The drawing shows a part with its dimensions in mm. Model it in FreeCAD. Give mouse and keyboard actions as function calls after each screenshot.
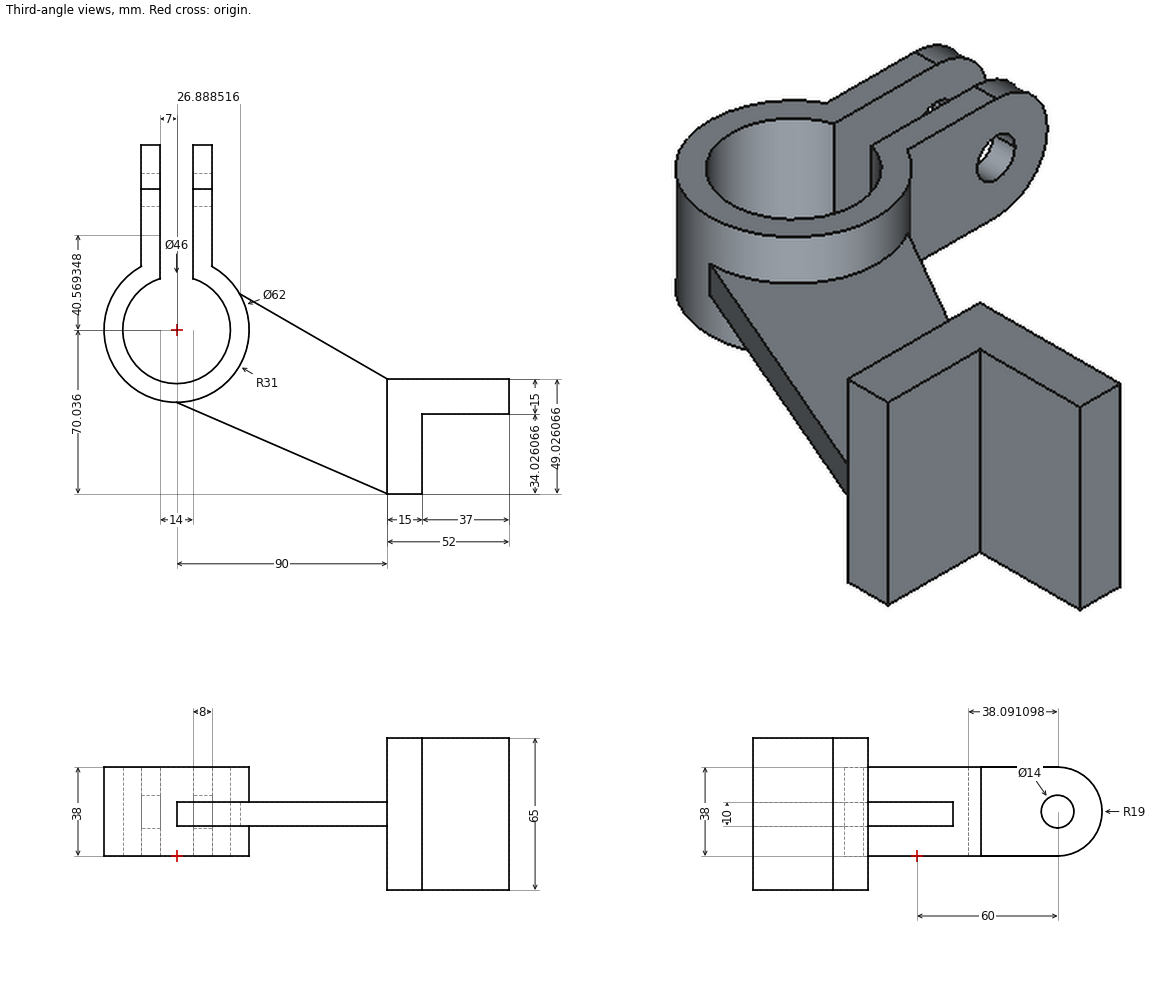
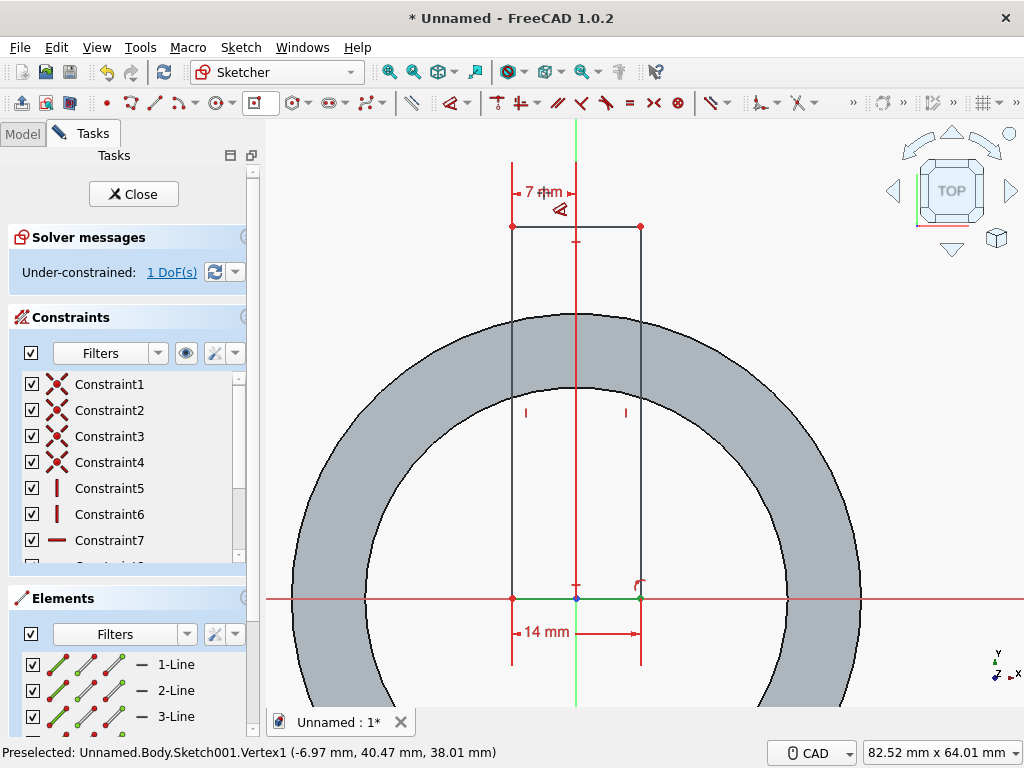
click(512, 339)
click(478, 413)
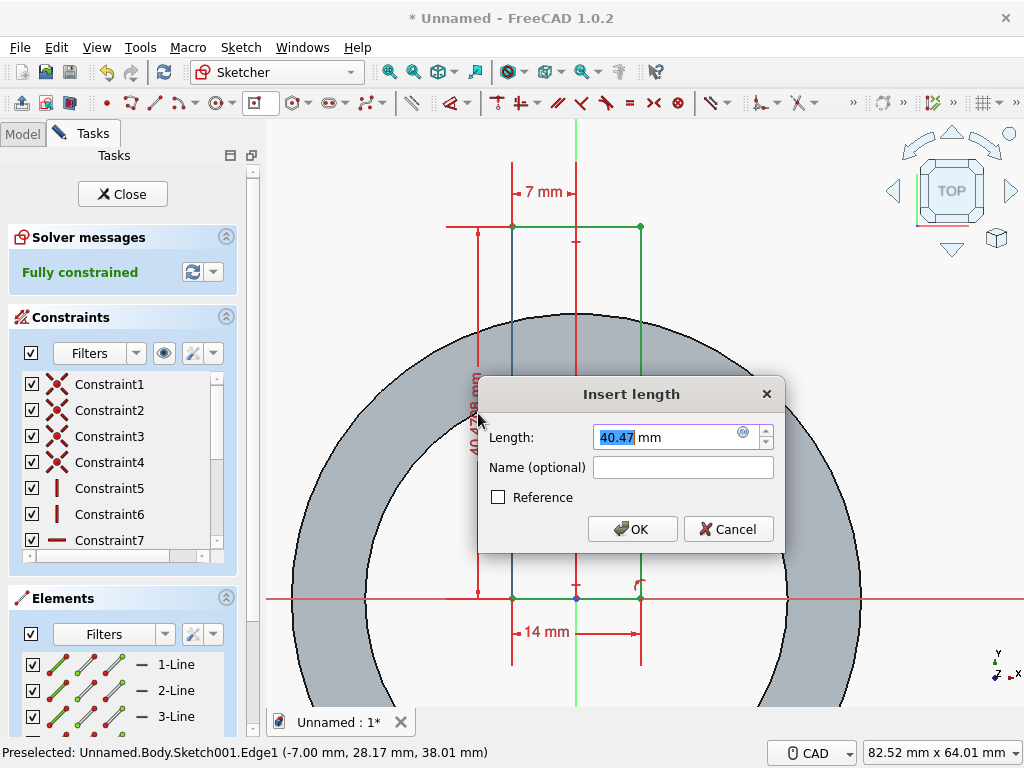
text(40.569348)
key(Return)
key(Escape)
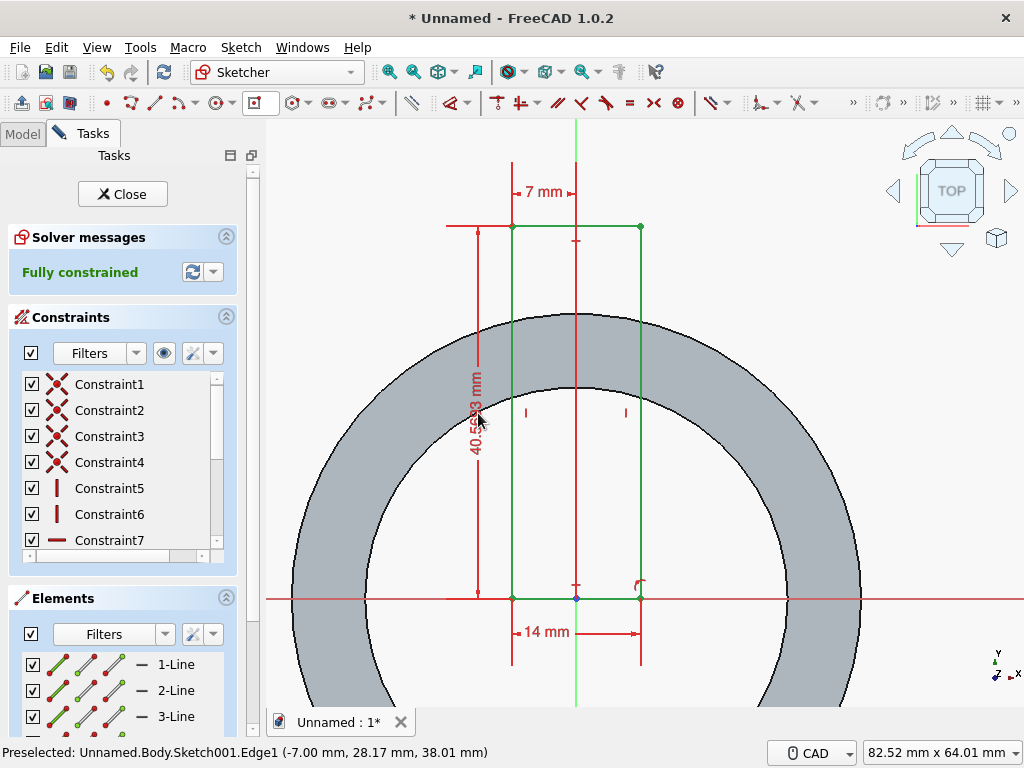
click(123, 194)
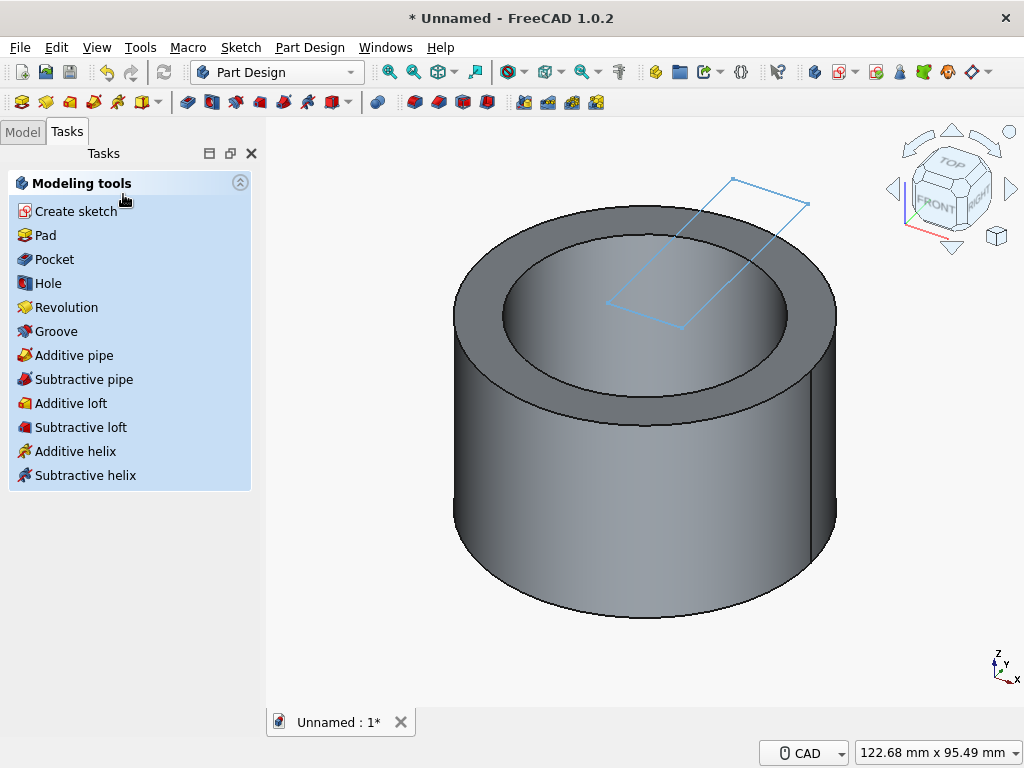
click(188, 102)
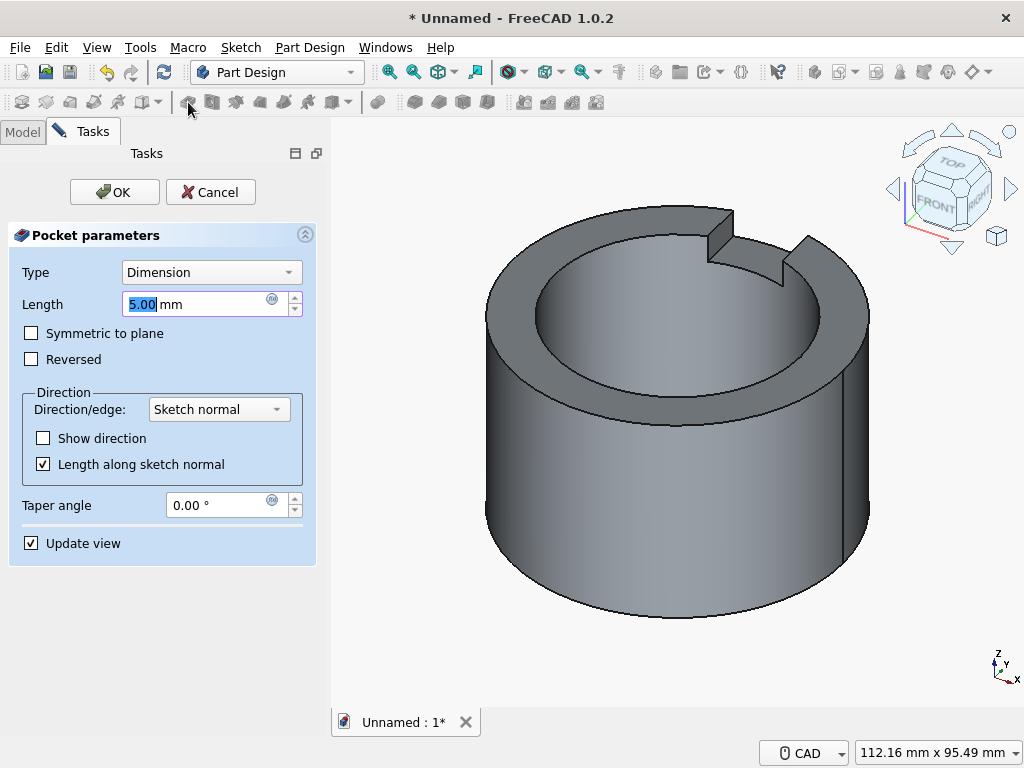
text(38)
key(Tab)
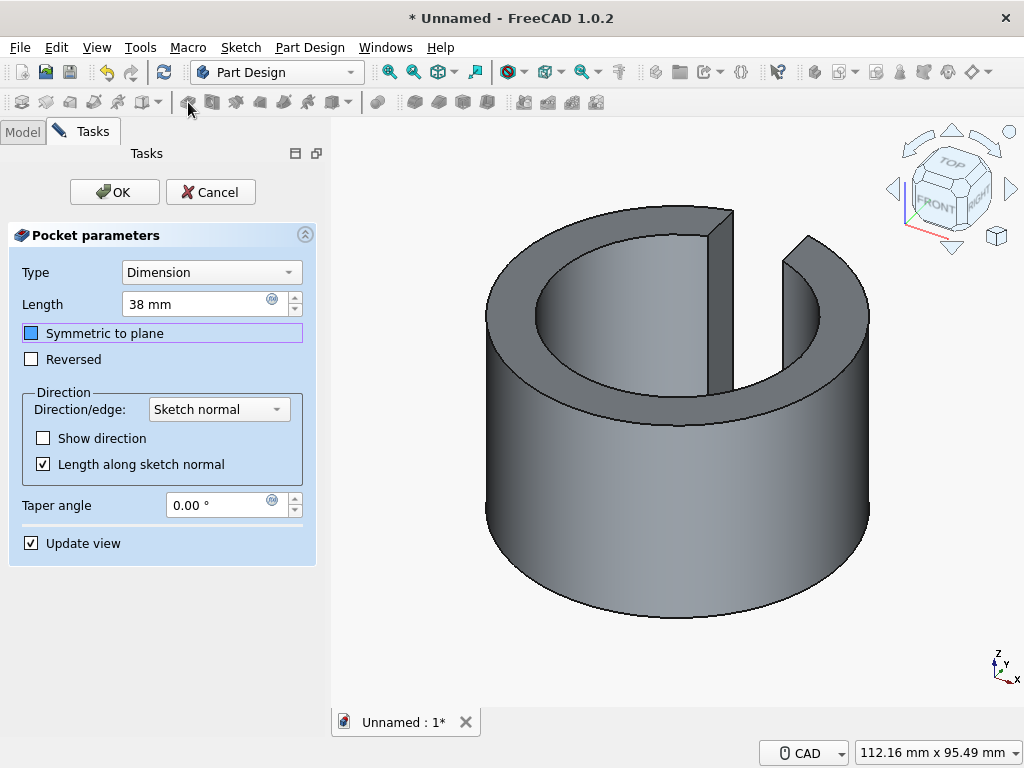
click(115, 192)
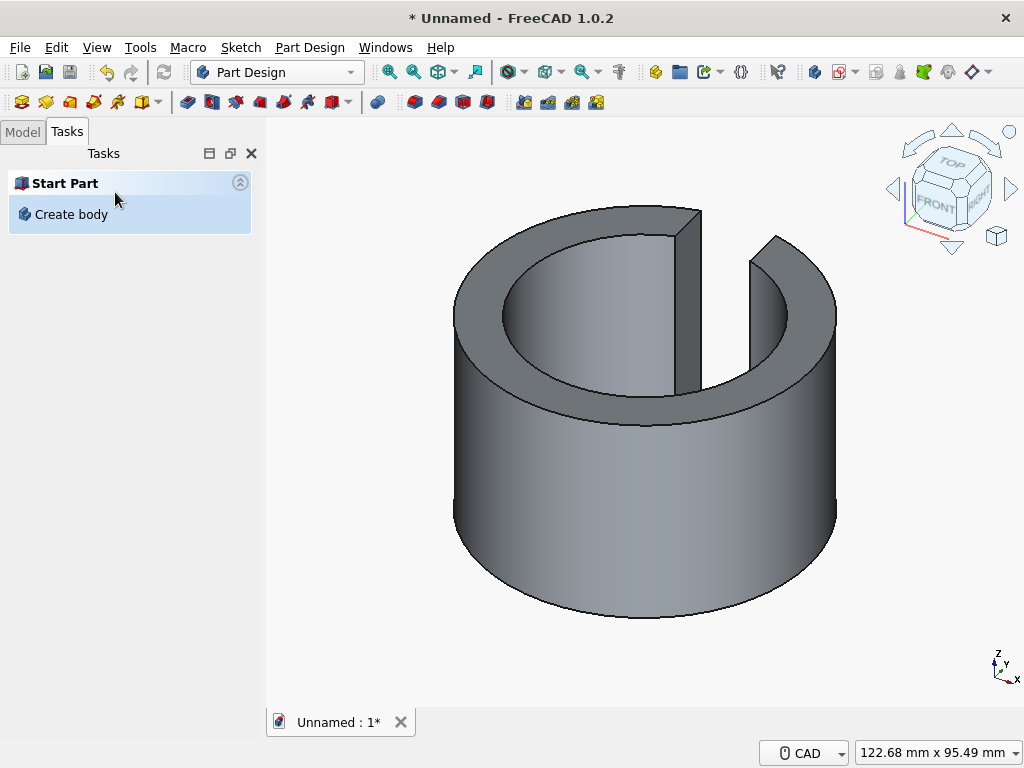
click(23, 131)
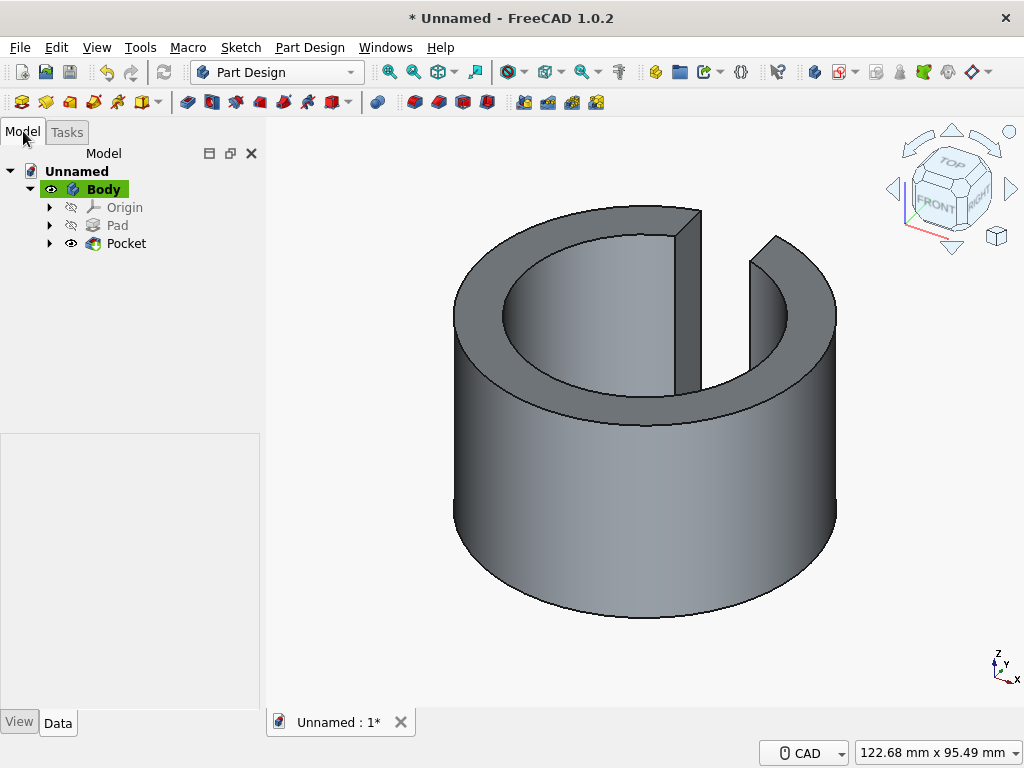
click(50, 207)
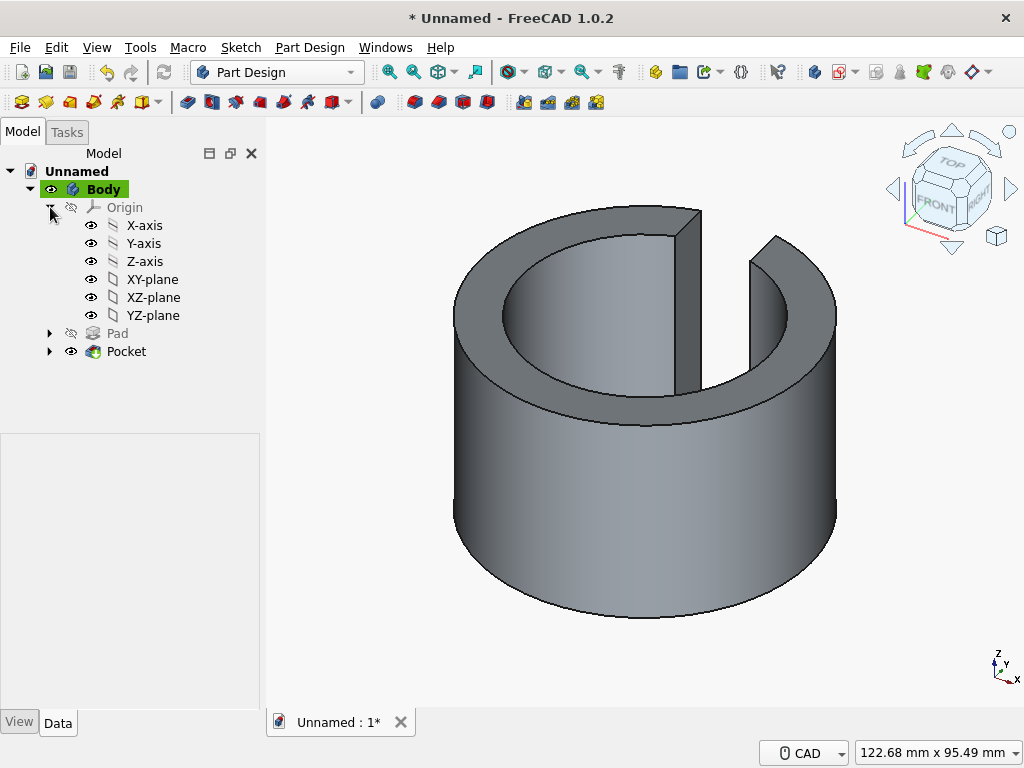
click(136, 315)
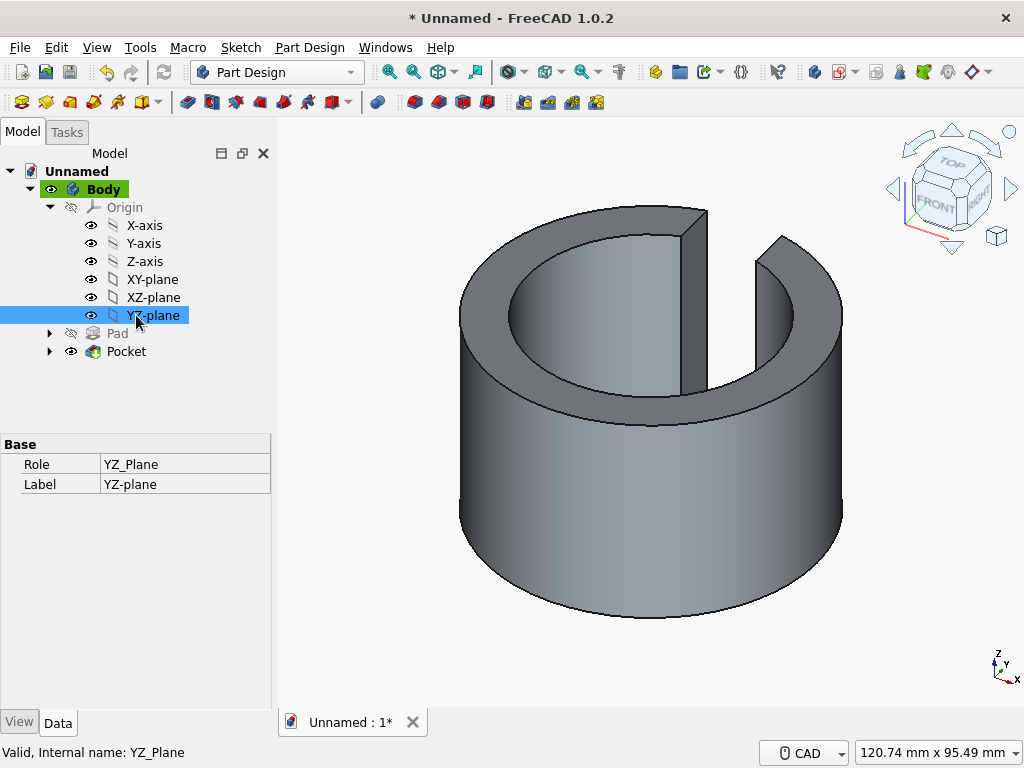
click(972, 72)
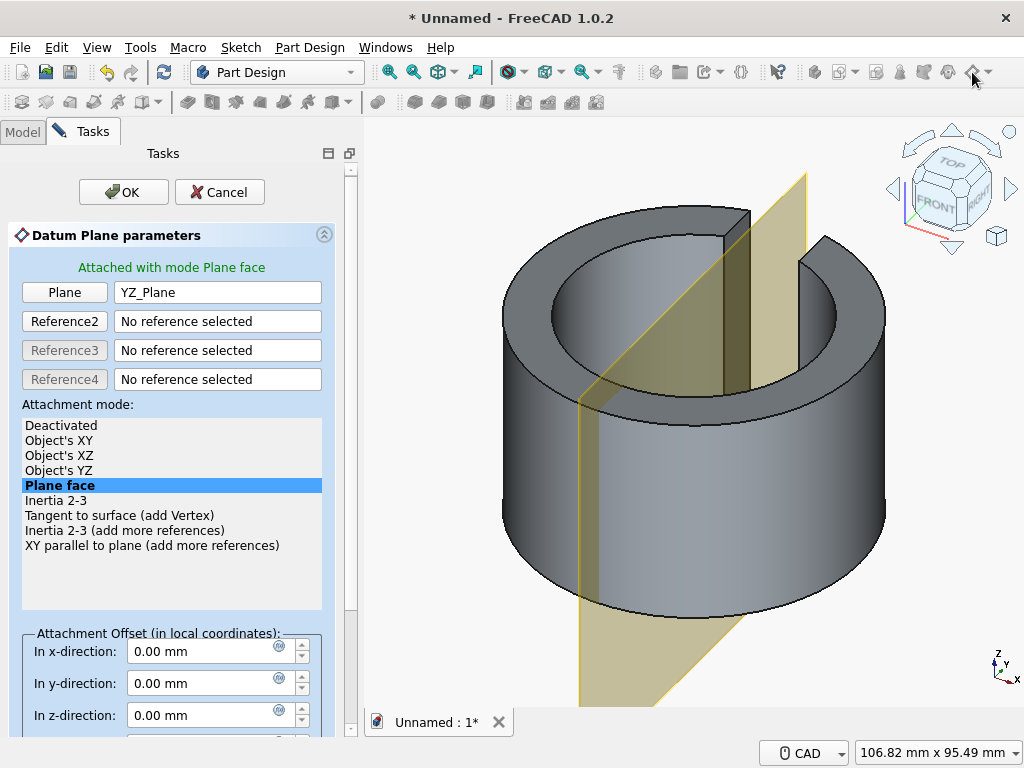
triple_click(210, 715)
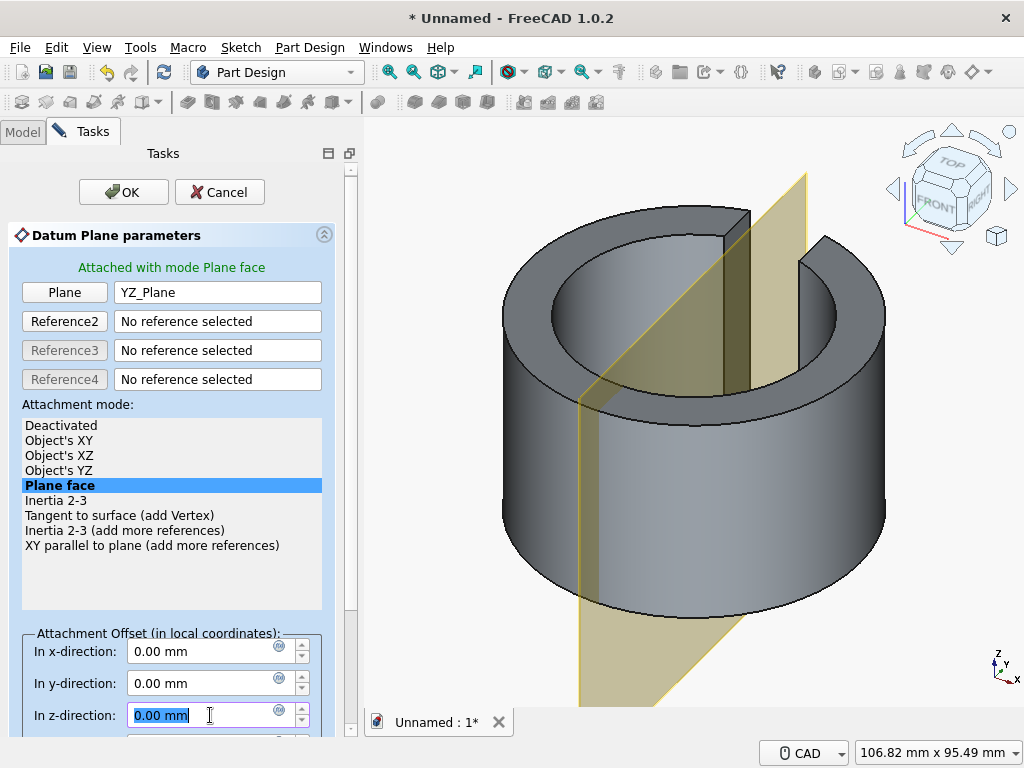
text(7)
key(Tab)